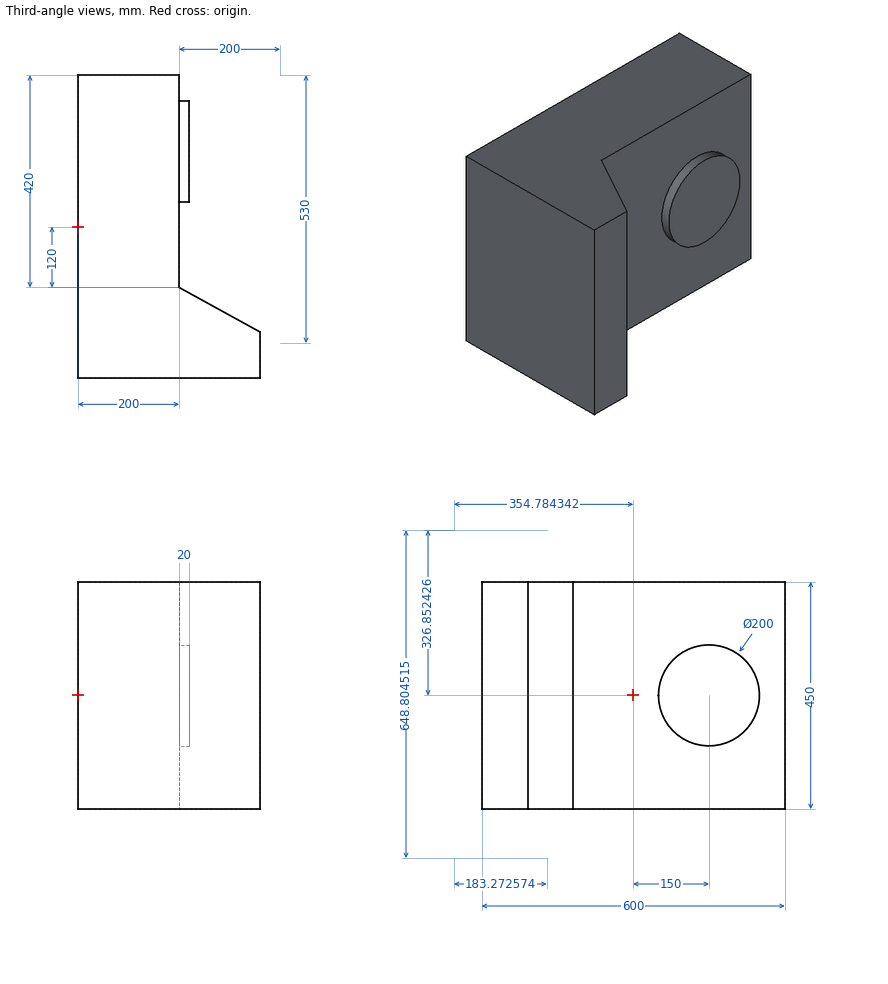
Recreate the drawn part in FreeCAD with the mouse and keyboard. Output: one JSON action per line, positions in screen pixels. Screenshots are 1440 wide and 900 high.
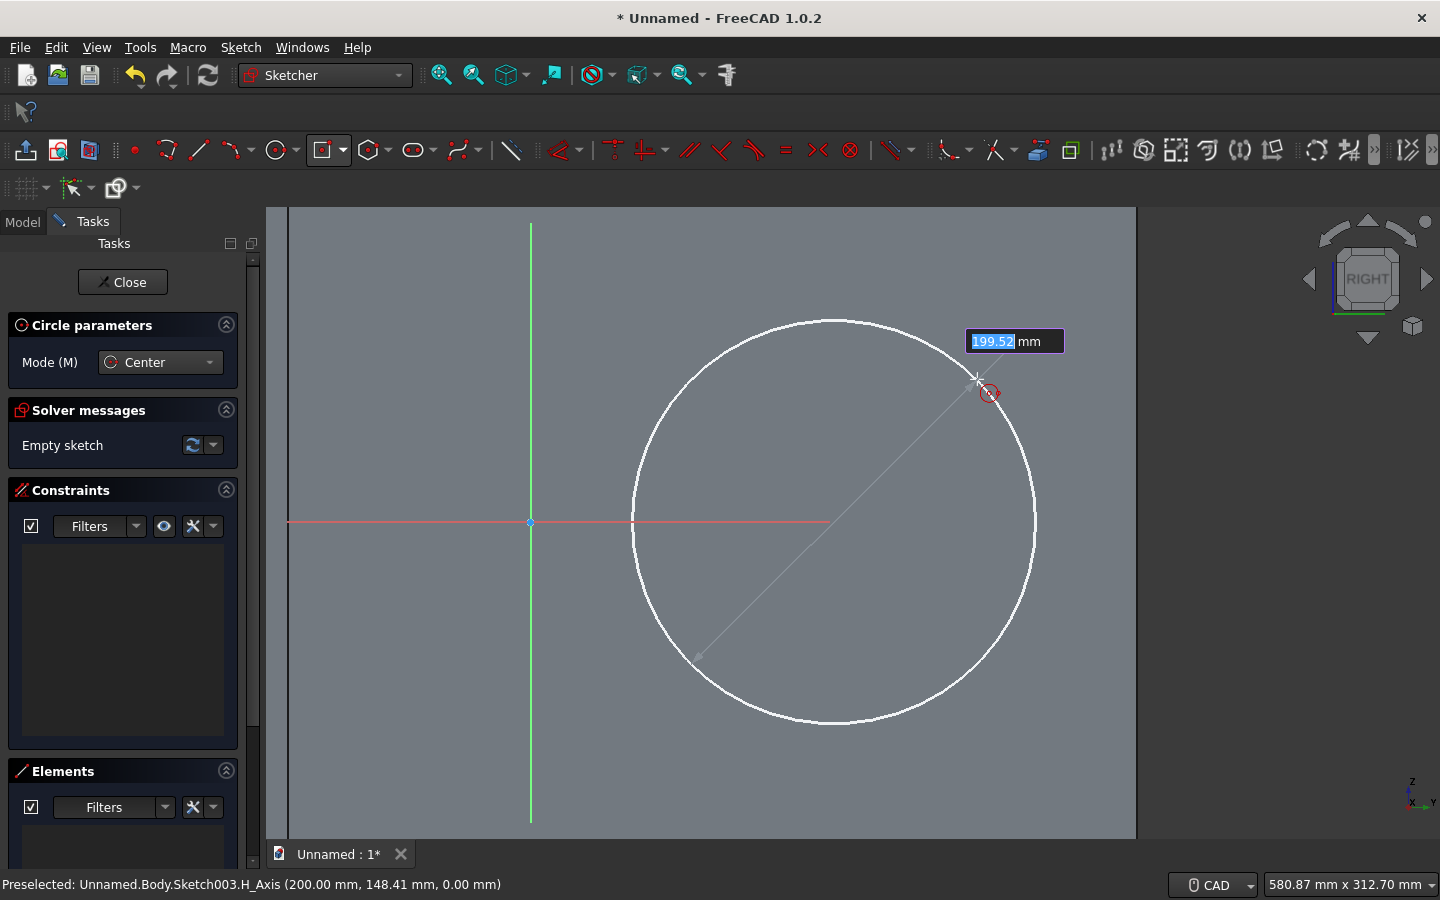
{"action": "type", "text": "200"}
{"action": "key", "text": "Return"}
{"action": "key", "text": "Escape"}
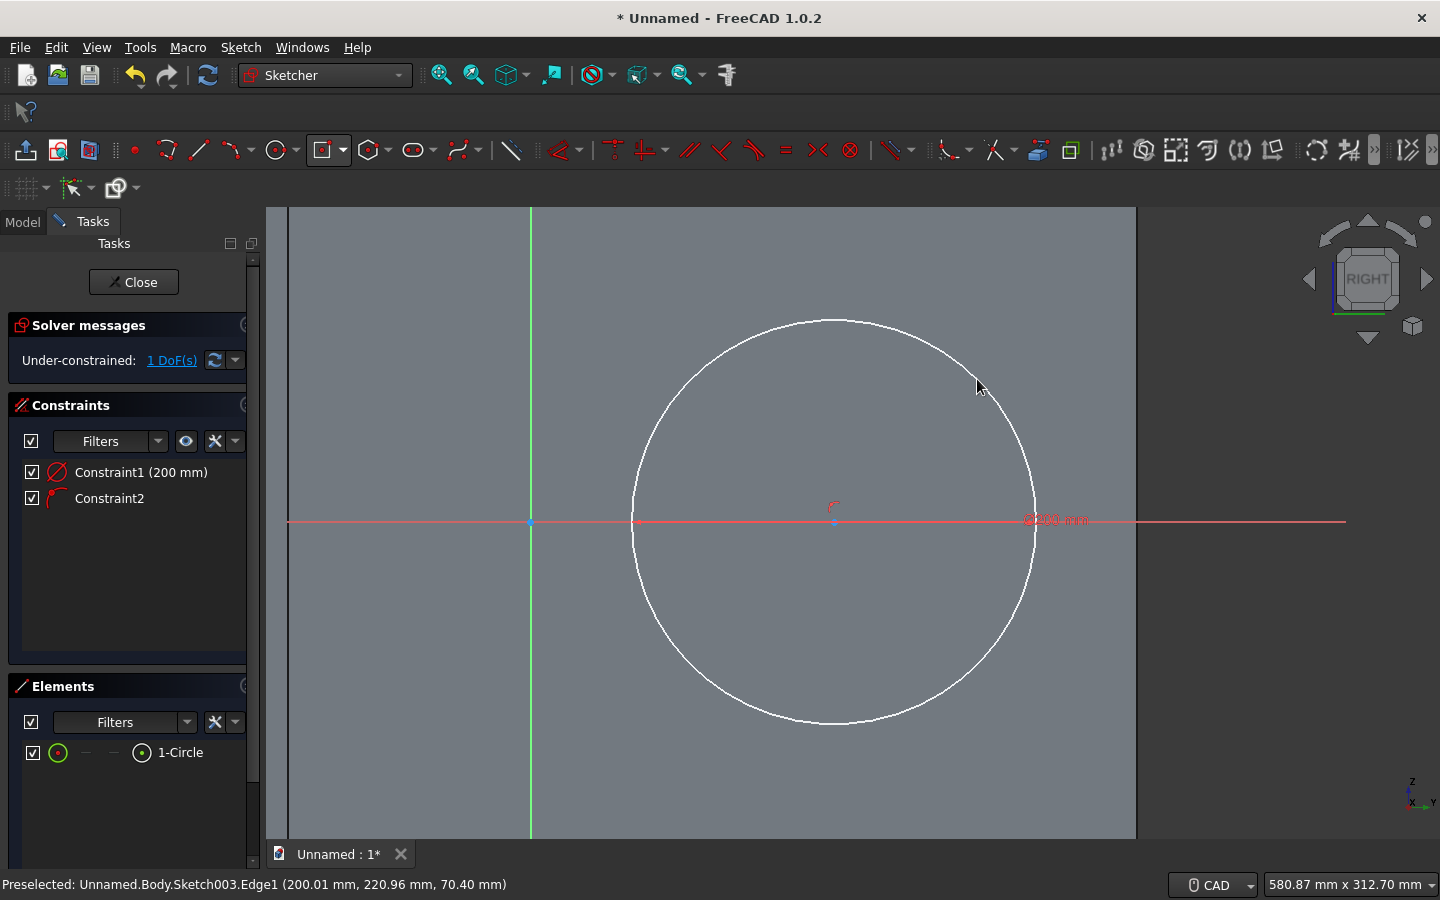
{"action": "key", "text": "d"}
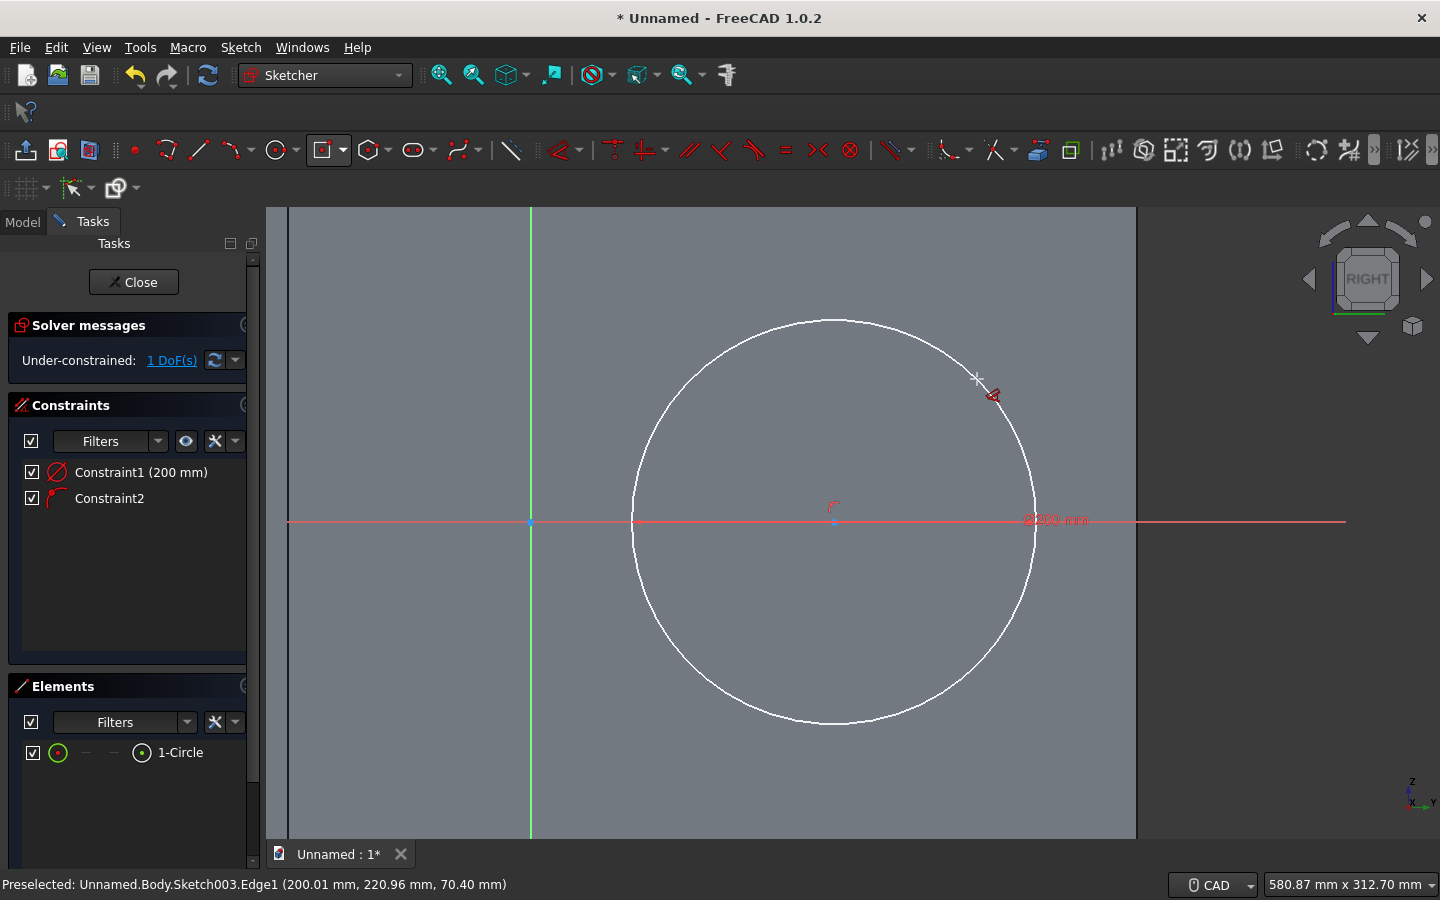
{"action": "left_click", "coordinate": [834, 522]}
{"action": "left_click", "coordinate": [682, 556]}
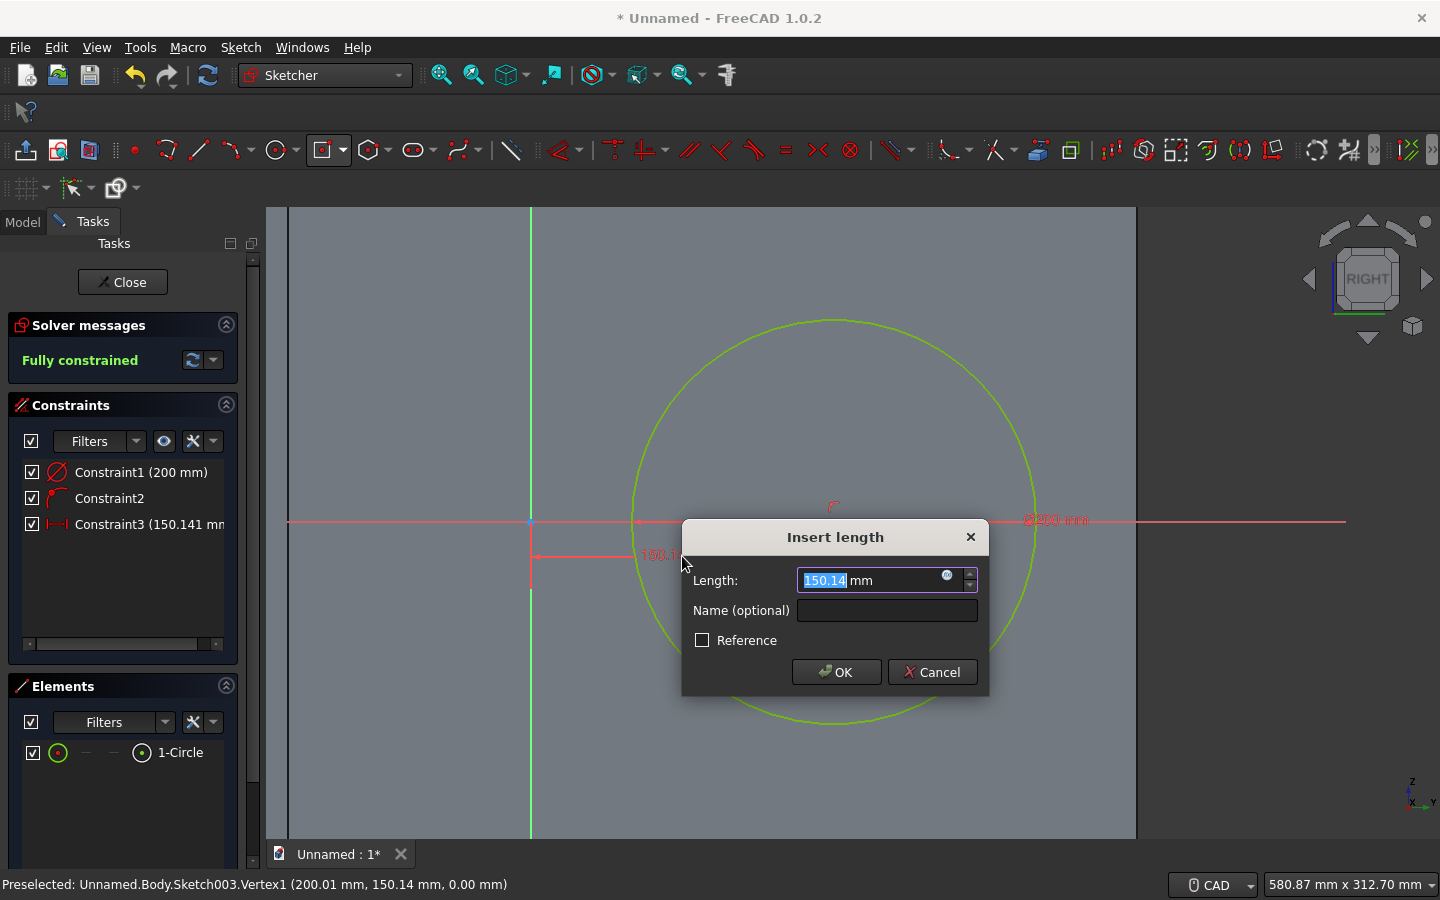
{"action": "type", "text": "150"}
{"action": "key", "text": "Return"}
{"action": "key", "text": "Escape"}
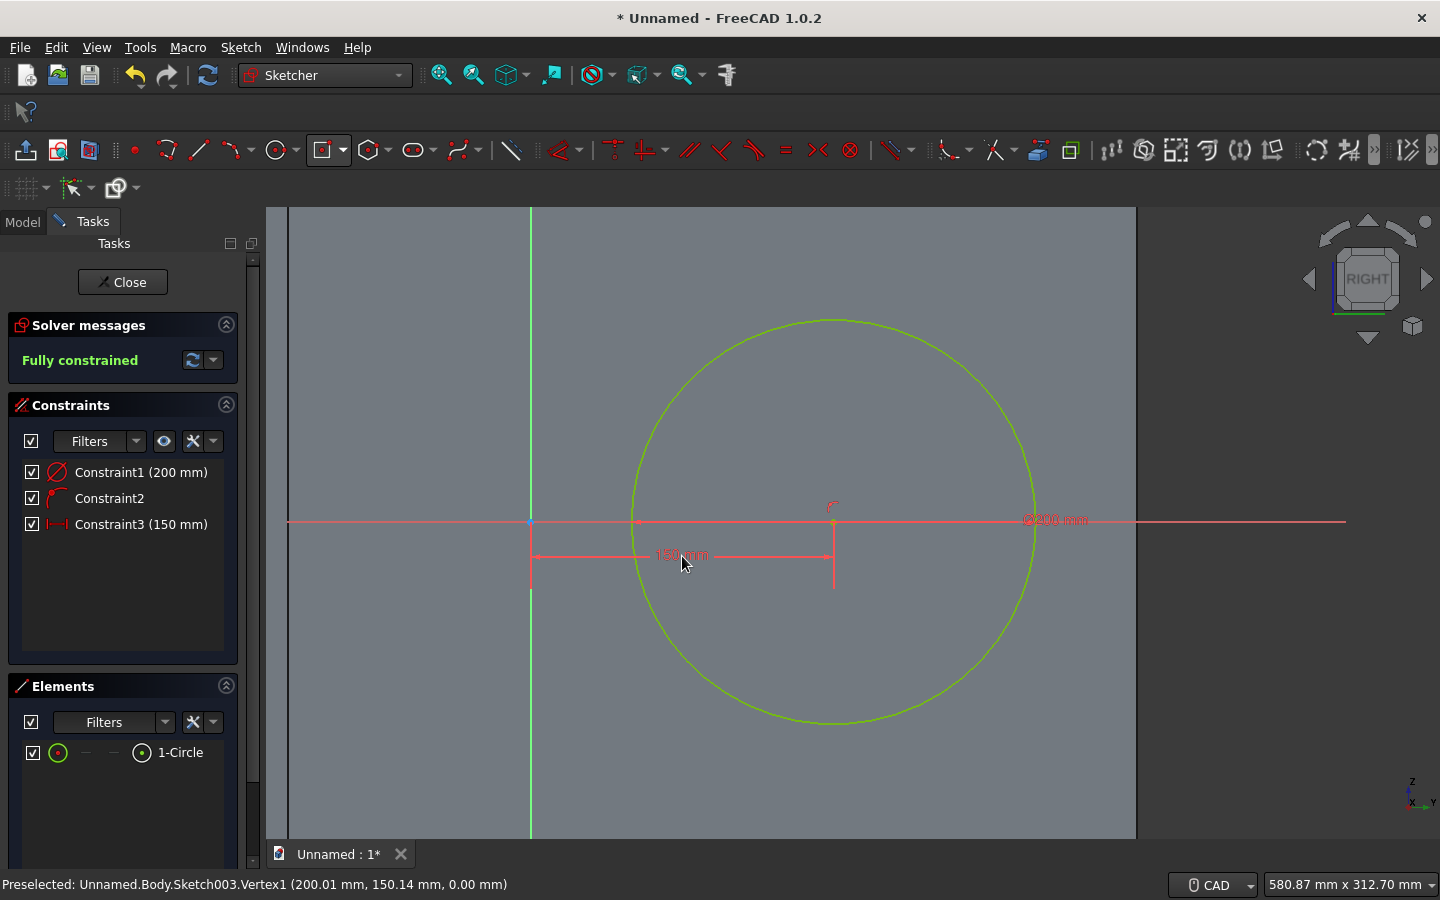
{"action": "left_click", "coordinate": [123, 282]}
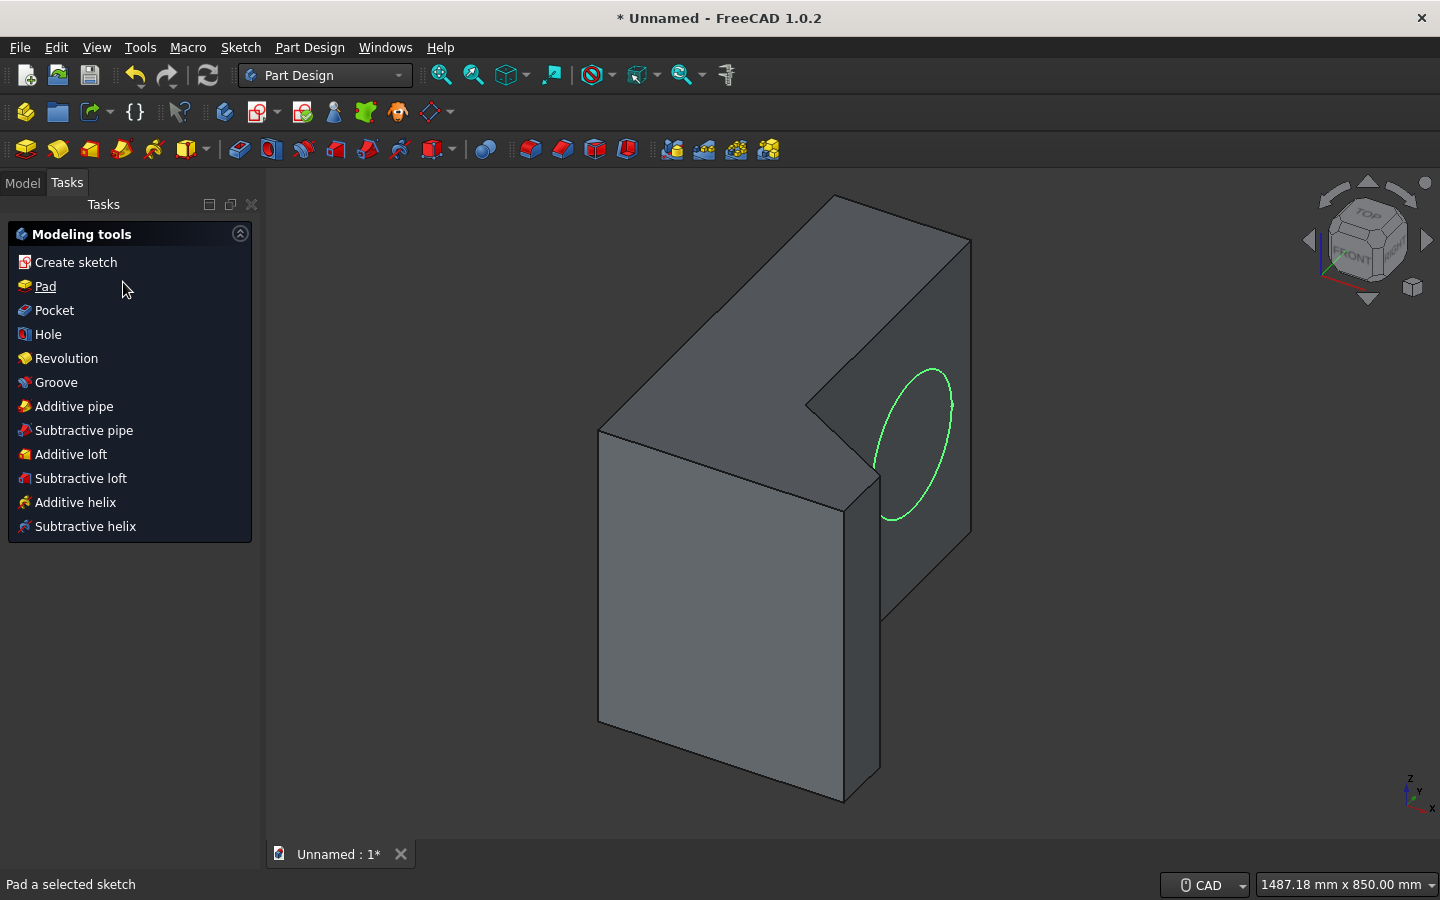
{"action": "left_click", "coordinate": [26, 150]}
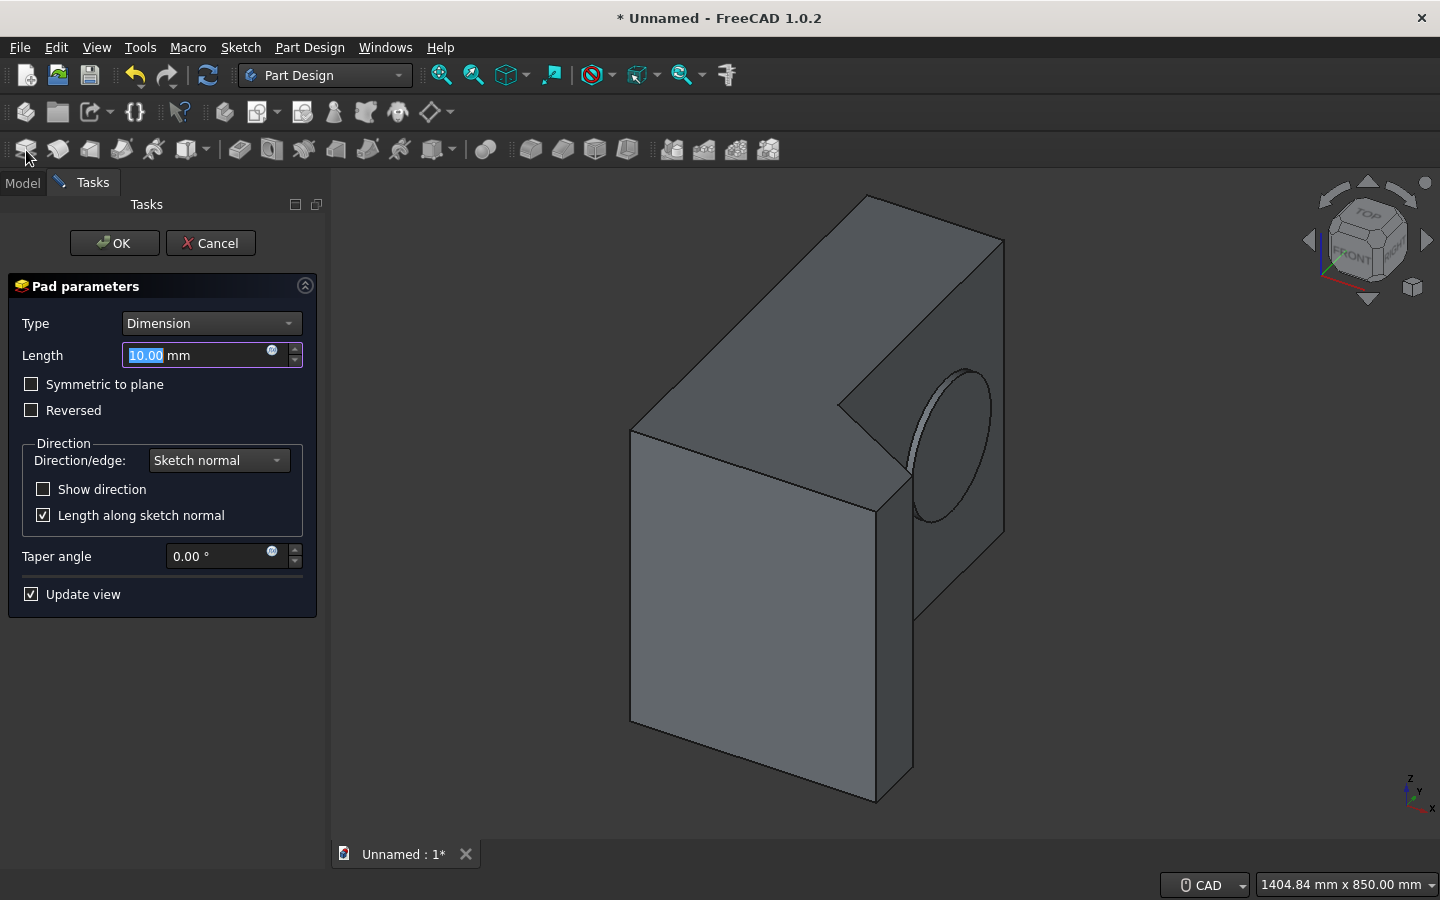
{"action": "type", "text": "20"}
{"action": "key", "text": "Tab"}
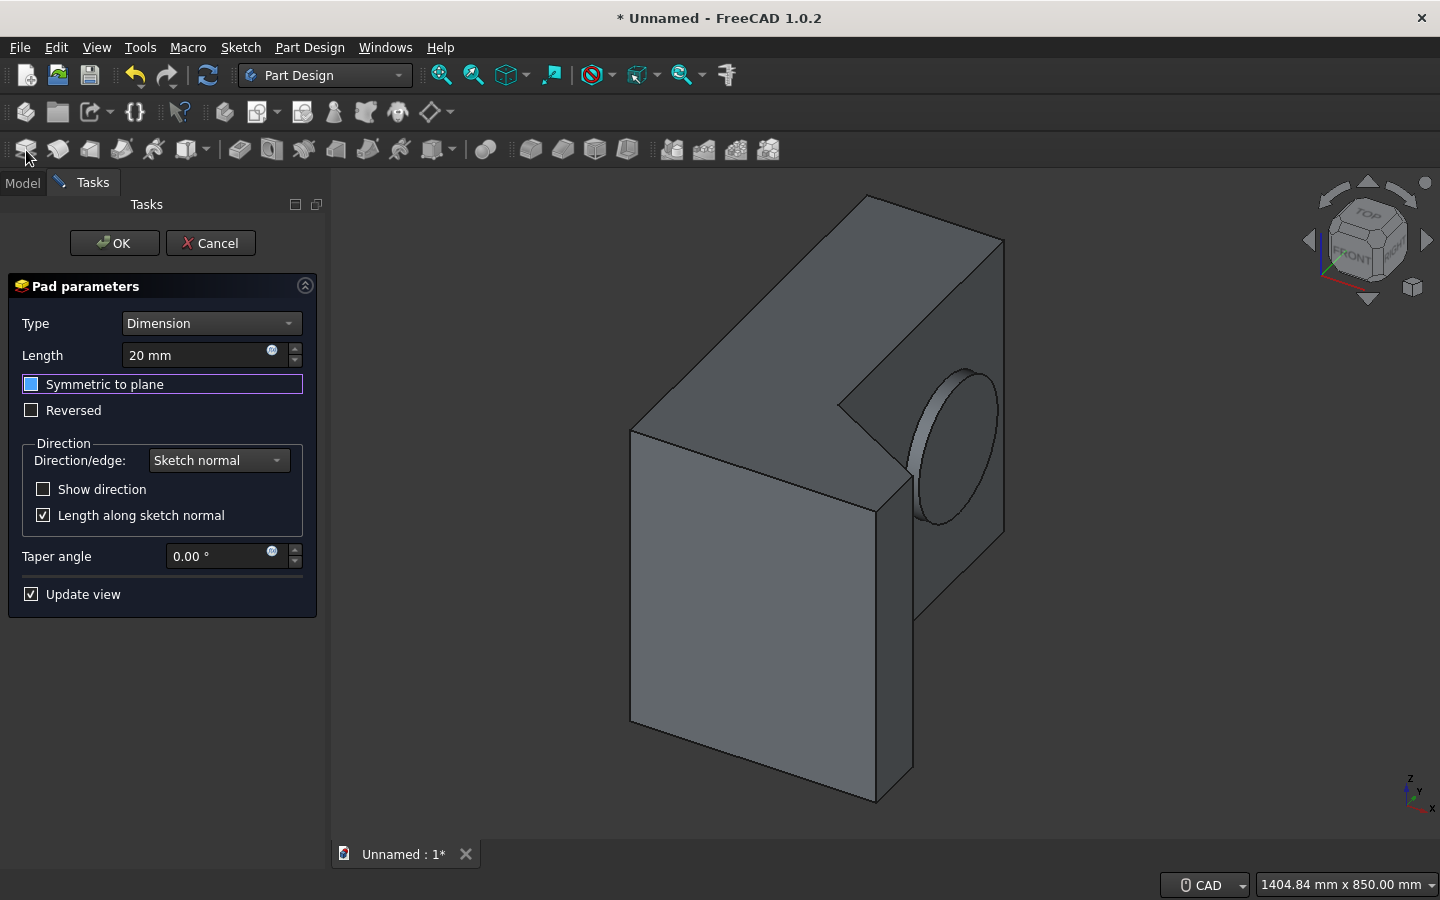
{"action": "left_click", "coordinate": [115, 243]}